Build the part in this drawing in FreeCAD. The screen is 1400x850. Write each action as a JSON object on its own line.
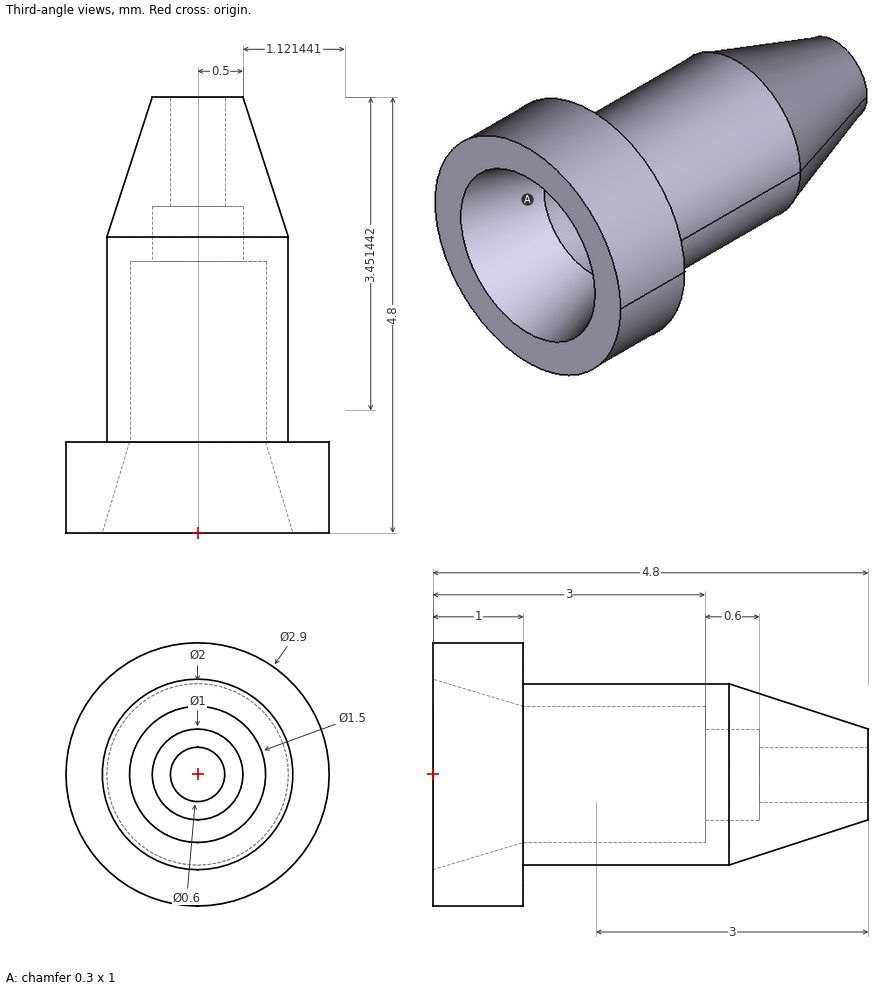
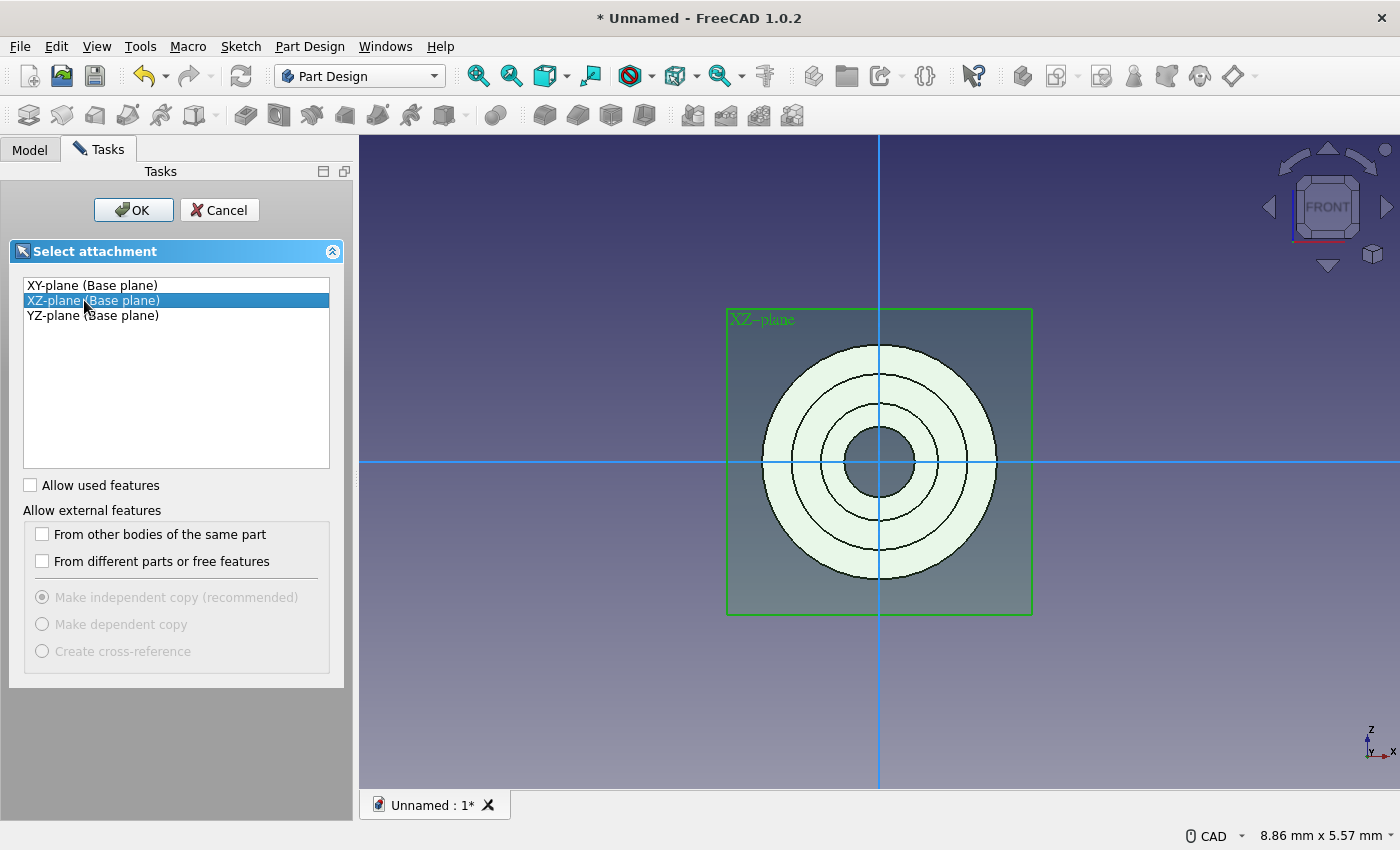
{"action": "left_click", "coordinate": [134, 210]}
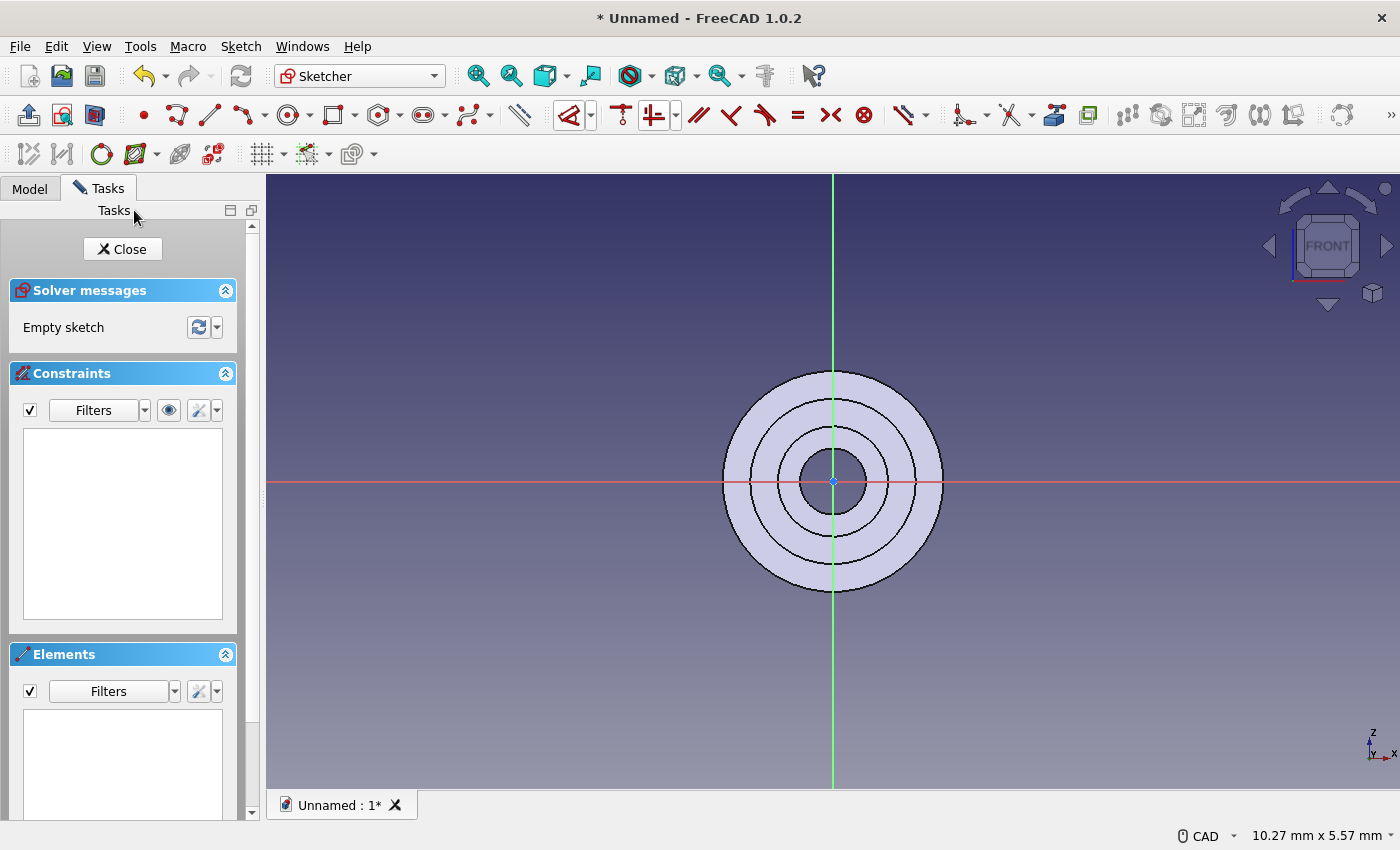
{"action": "left_click", "coordinate": [288, 116]}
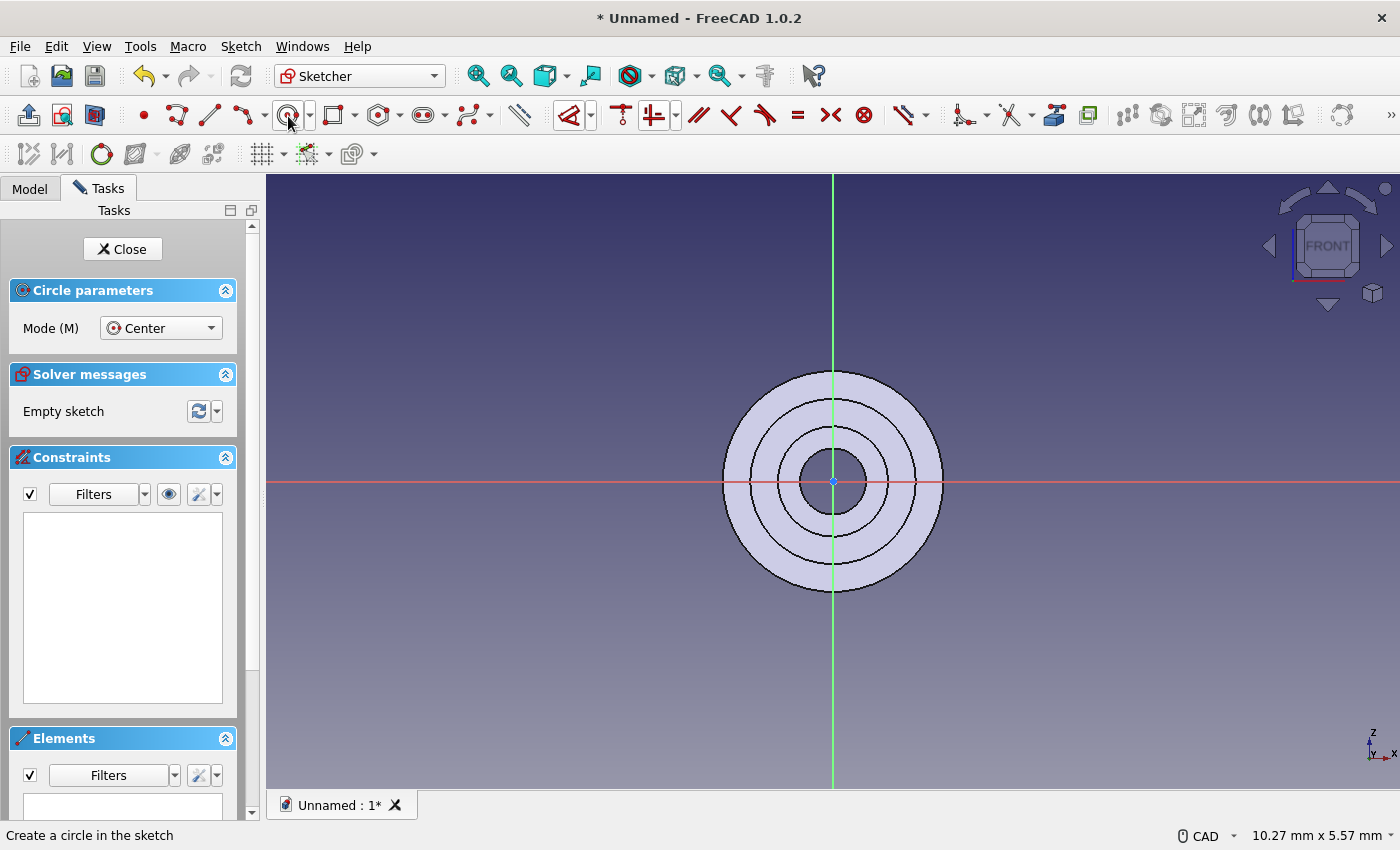
{"action": "left_click", "coordinate": [833, 482]}
{"action": "left_click", "coordinate": [946, 368]}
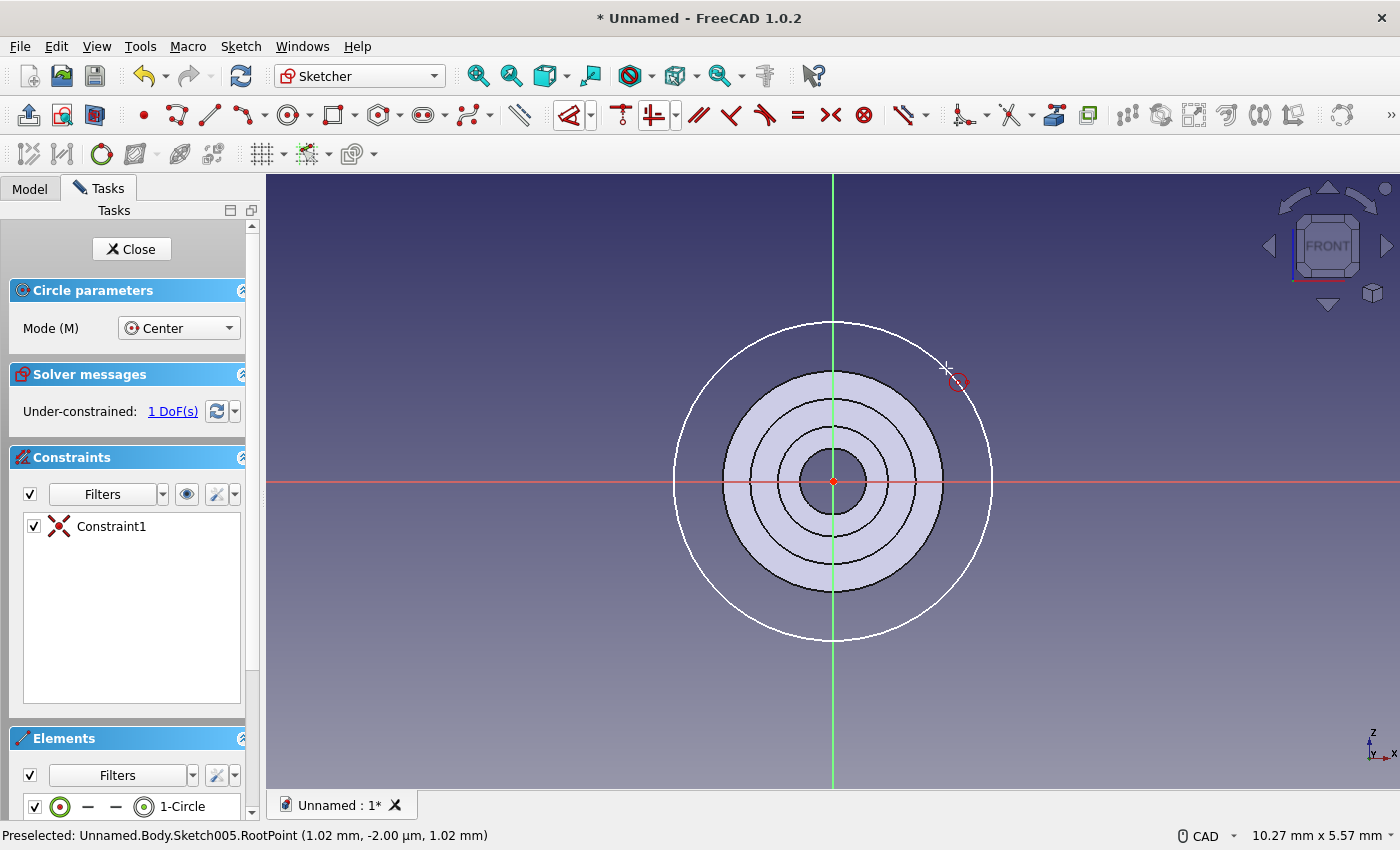
{"action": "left_click", "coordinate": [833, 482]}
{"action": "left_click", "coordinate": [911, 403]}
{"action": "key", "text": "Escape"}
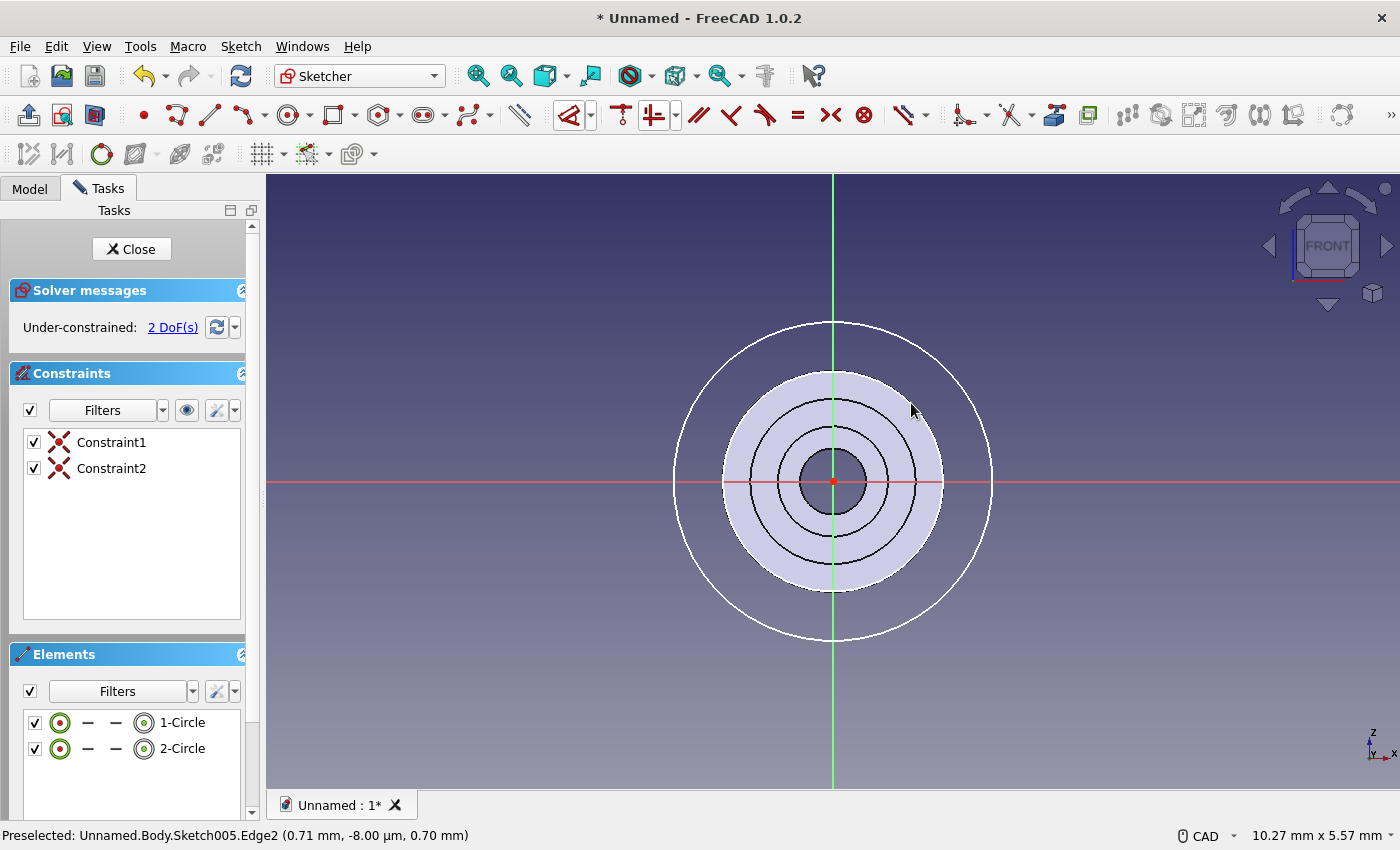
{"action": "left_click", "coordinate": [945, 368]}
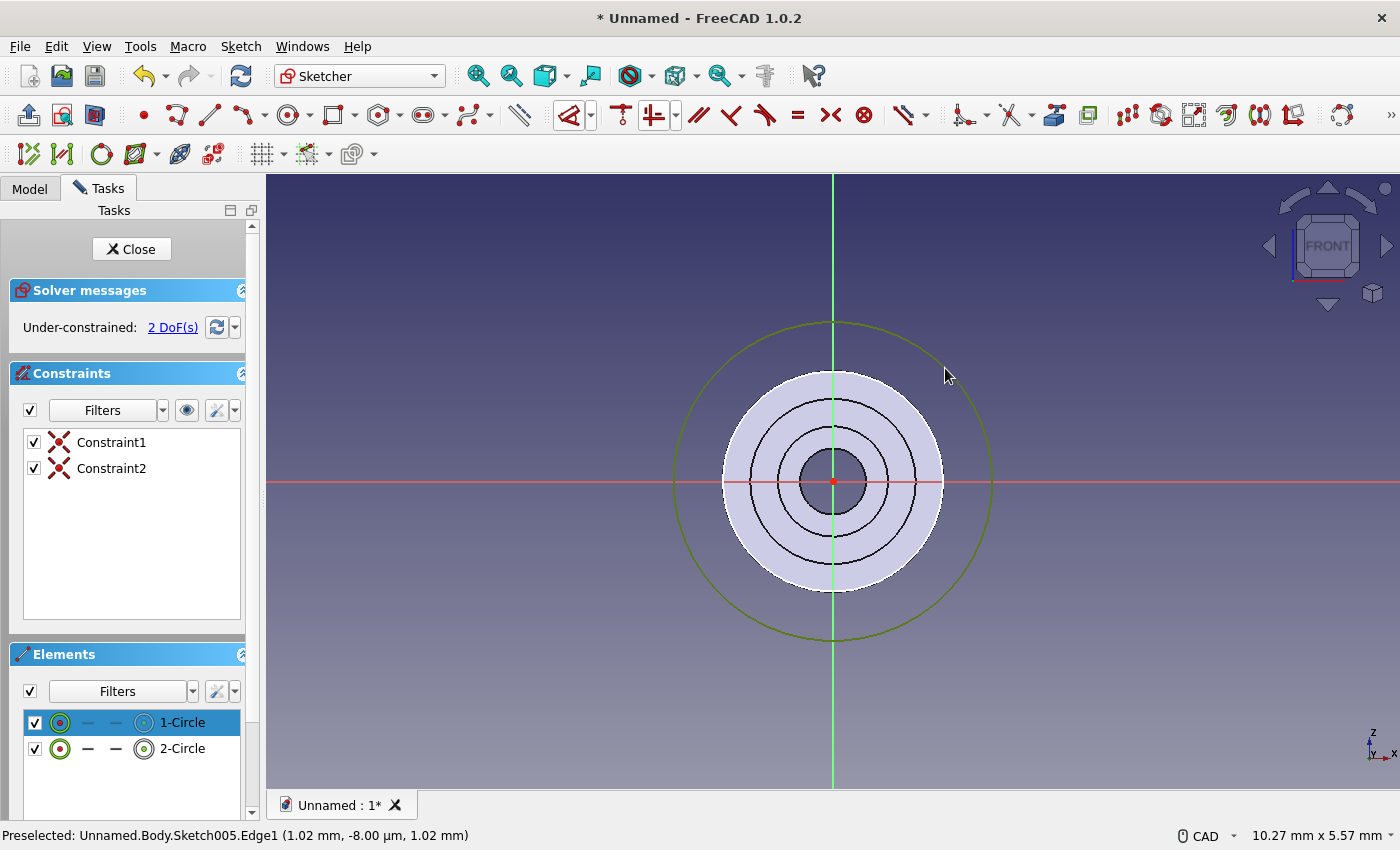
{"action": "left_click", "coordinate": [590, 116]}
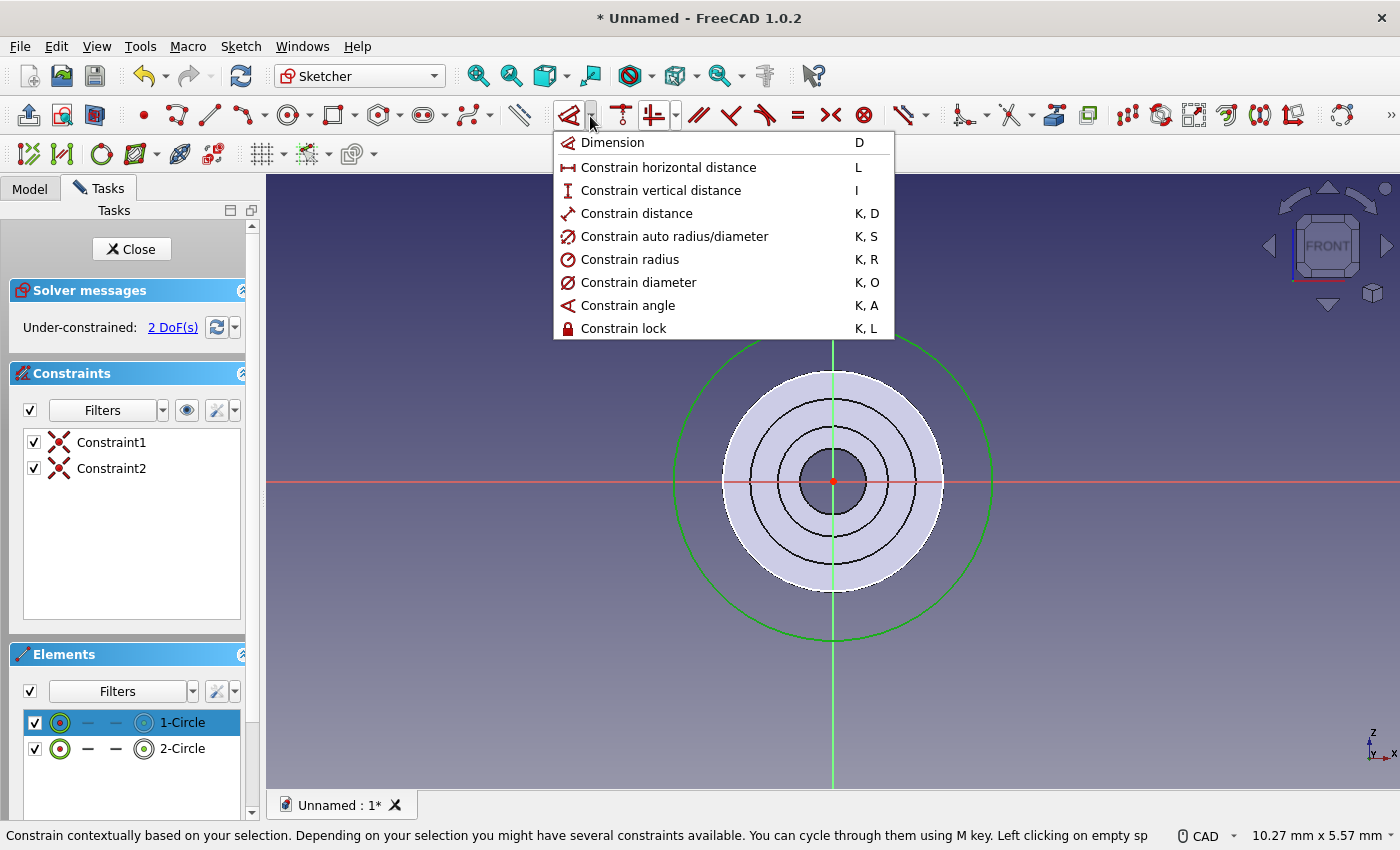
{"action": "left_click", "coordinate": [724, 282]}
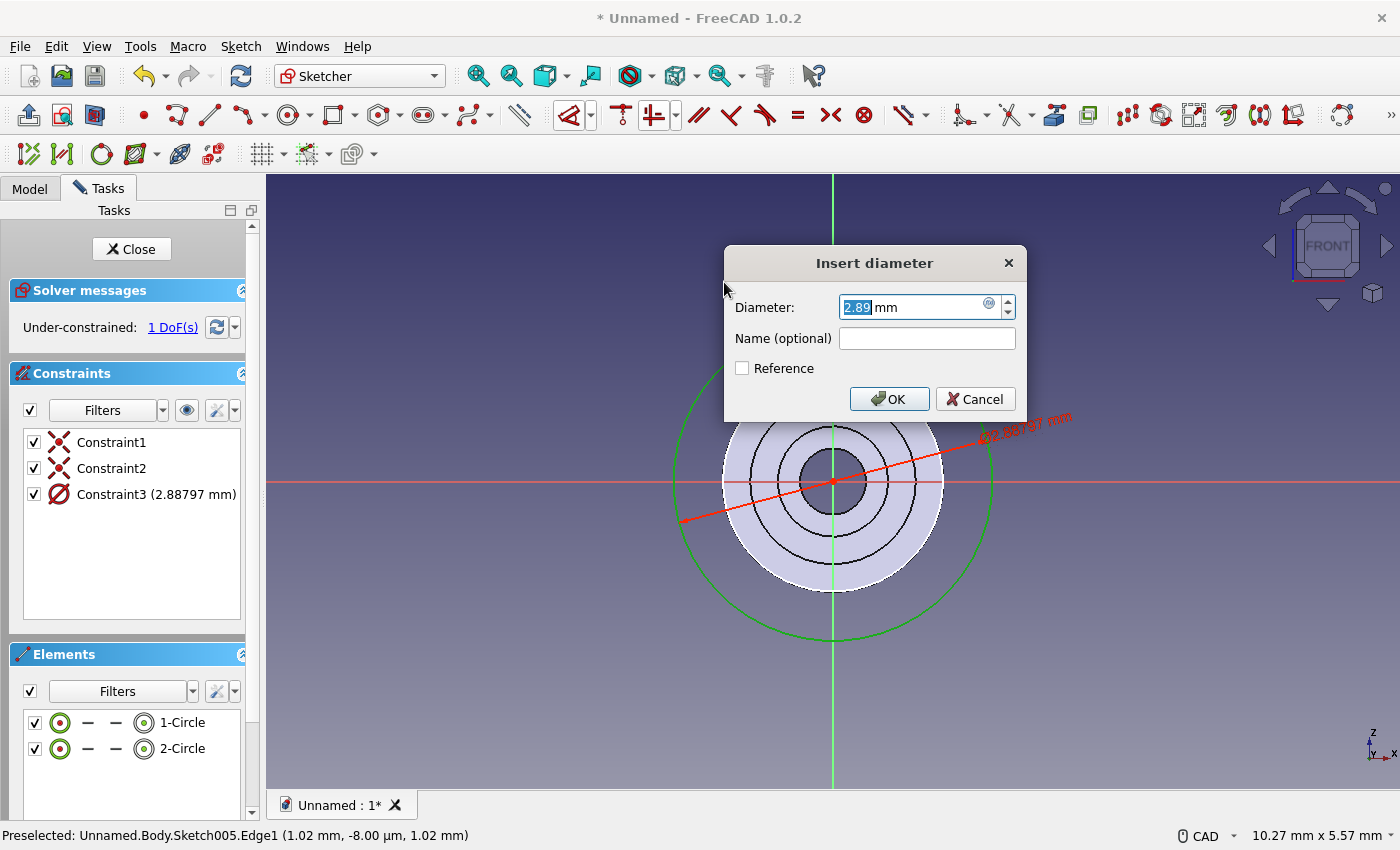
{"action": "type", "text": "2.9"}
{"action": "key", "text": "Return"}